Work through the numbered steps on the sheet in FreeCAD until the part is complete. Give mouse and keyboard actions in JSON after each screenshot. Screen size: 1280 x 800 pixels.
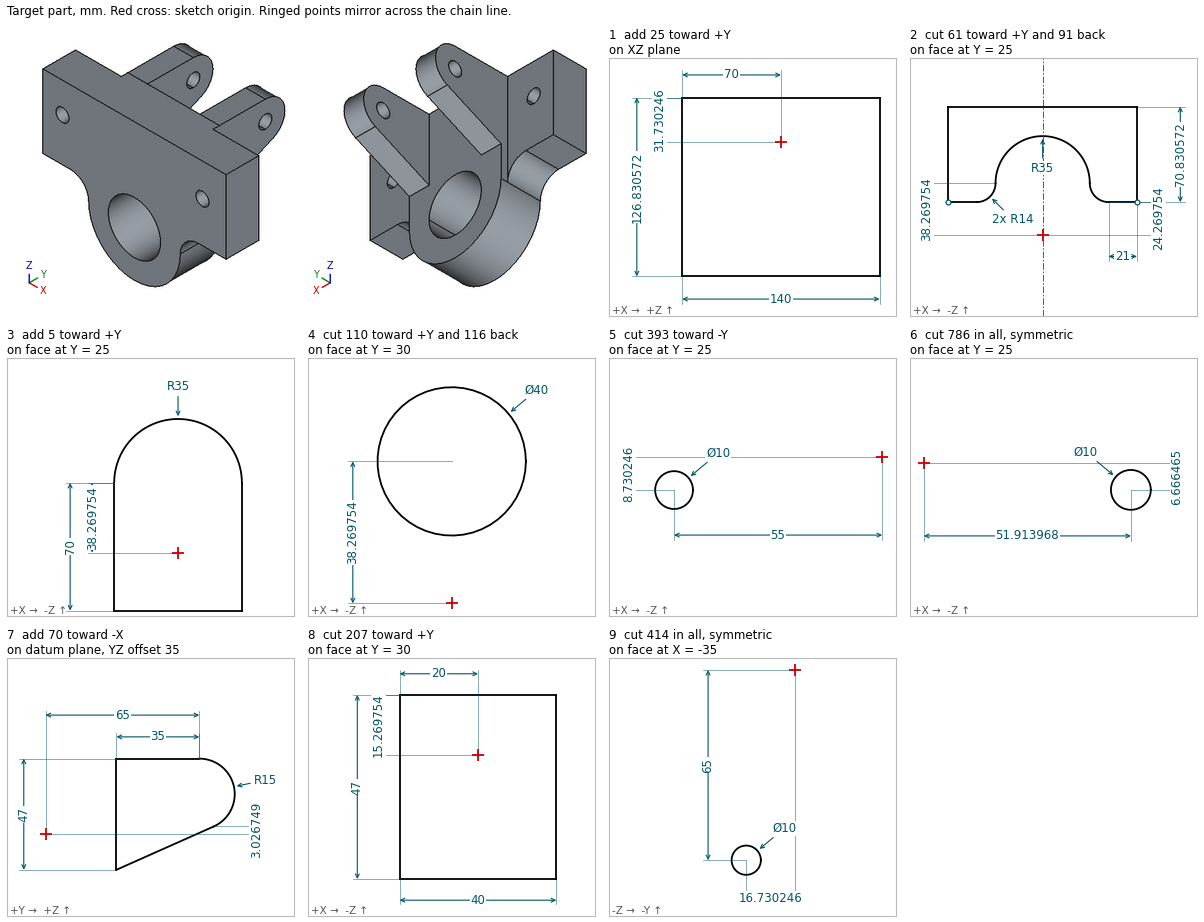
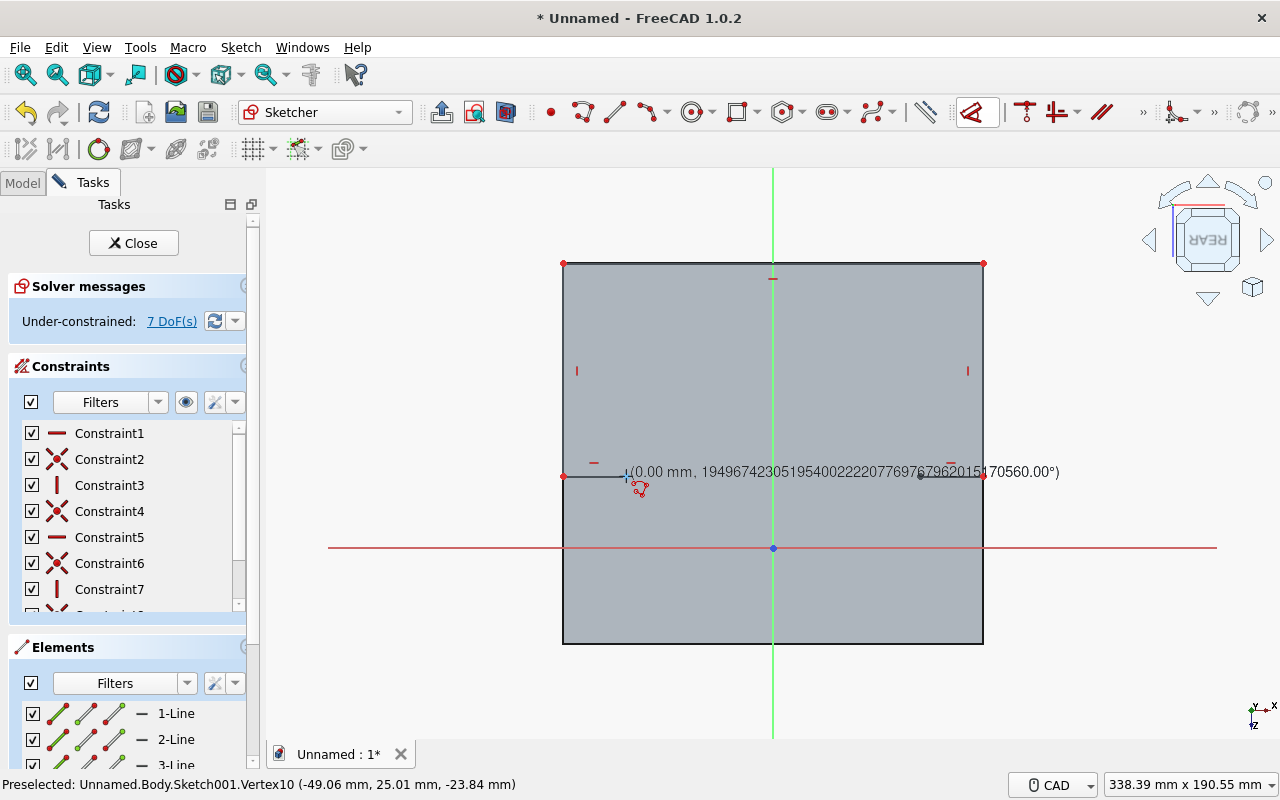
{"action": "left_click", "coordinate": [648, 112]}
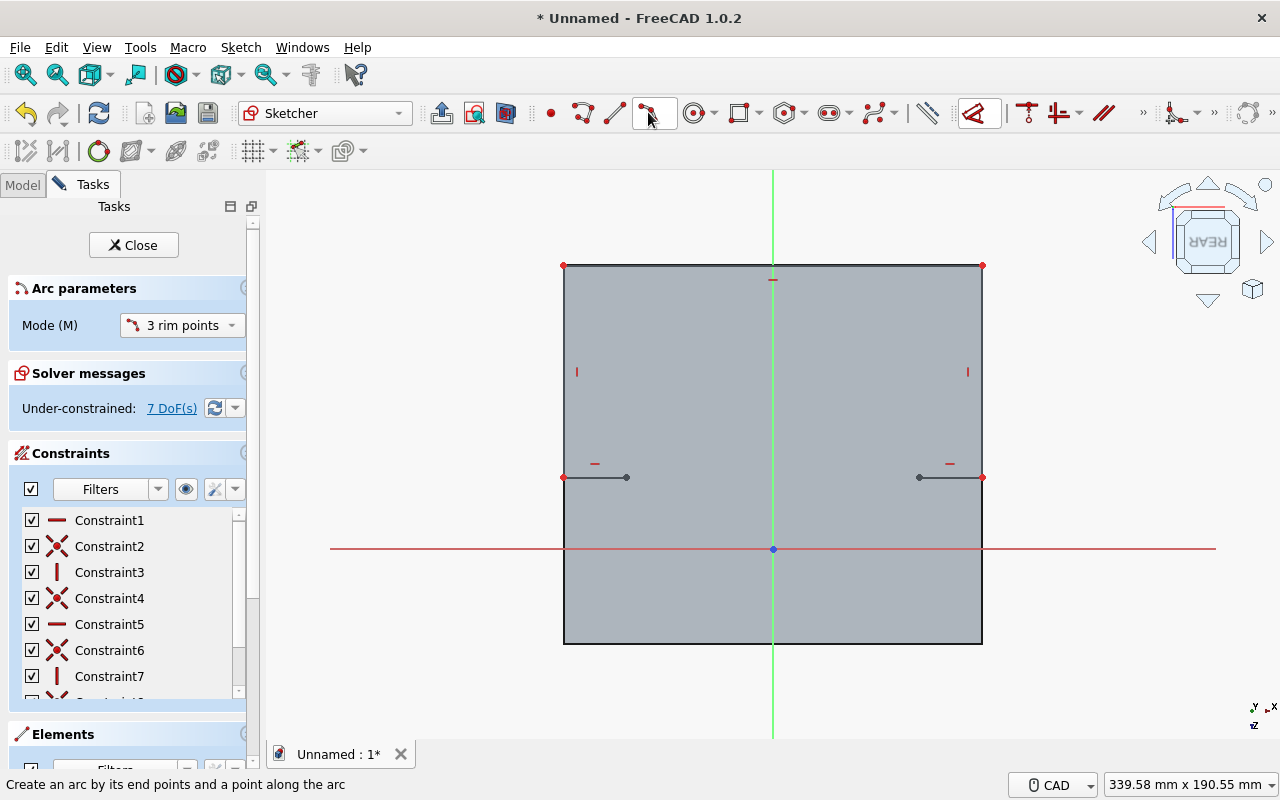
{"action": "left_click", "coordinate": [627, 478]}
{"action": "left_click", "coordinate": [668, 435]}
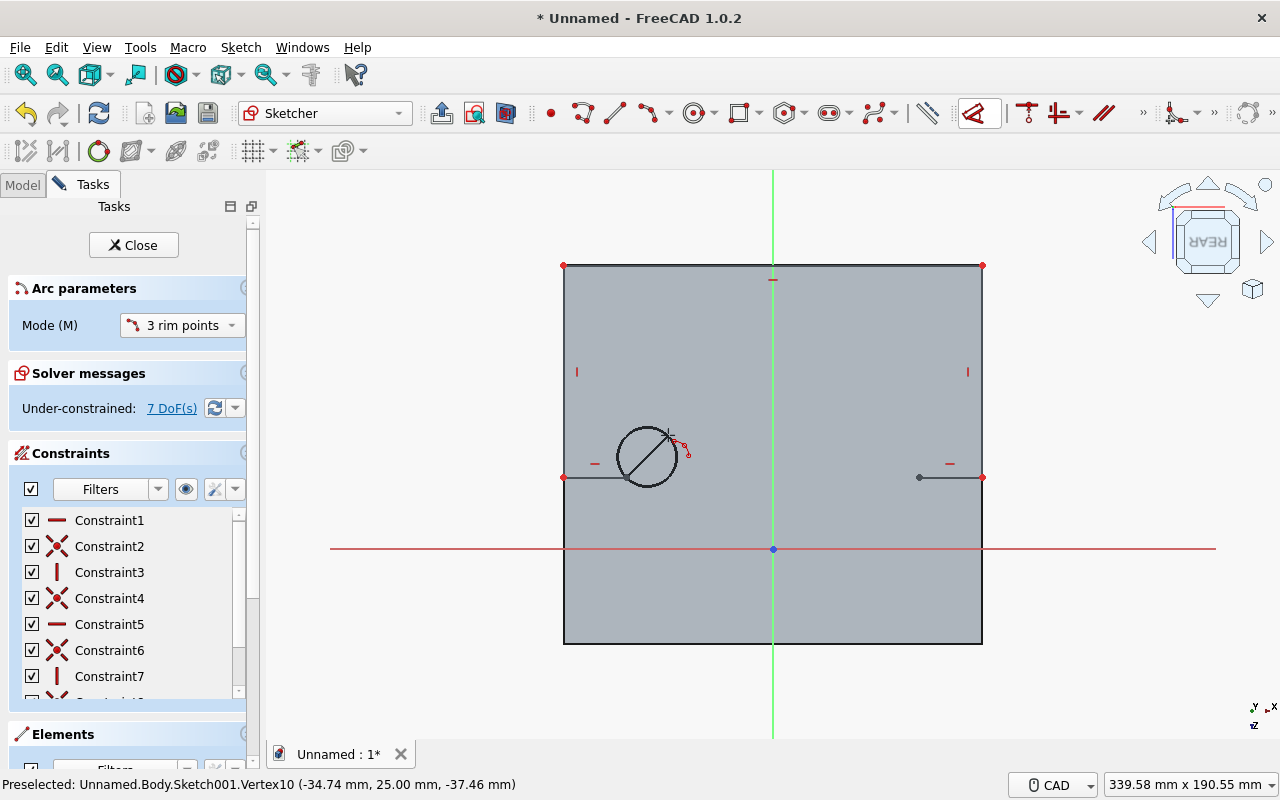
{"action": "scroll", "coordinate": [656, 464], "scroll_direction": "up", "scroll_amount": 2}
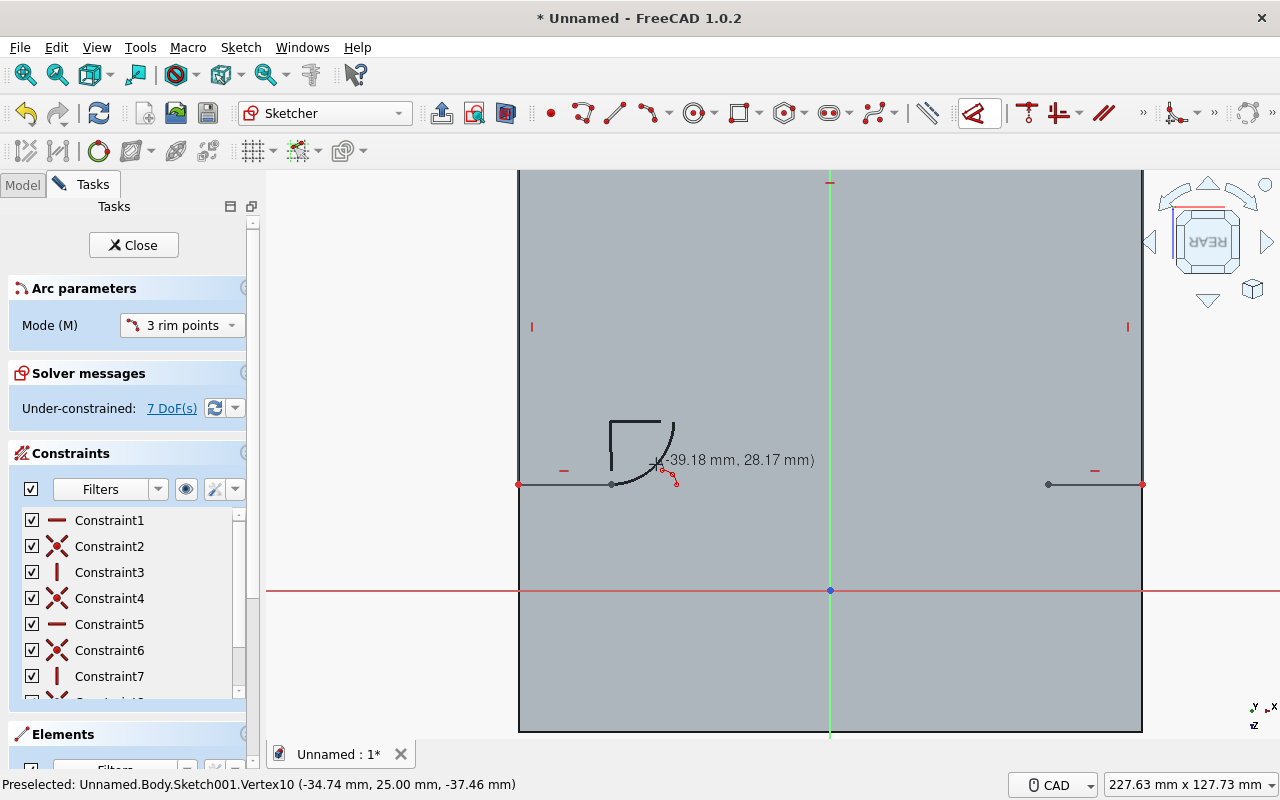
{"action": "left_click", "coordinate": [656, 464]}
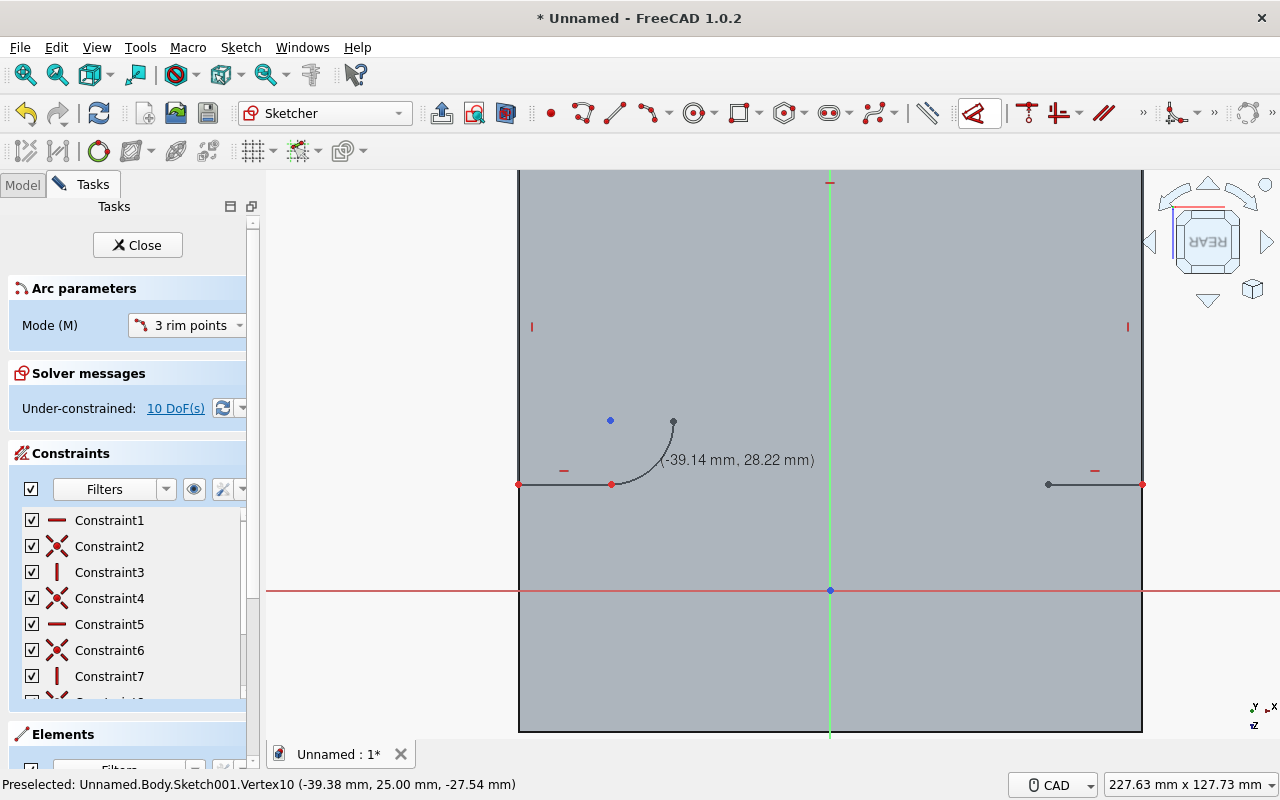
{"action": "left_click", "coordinate": [674, 422]}
{"action": "left_click", "coordinate": [986, 420]}
{"action": "left_click", "coordinate": [879, 272]}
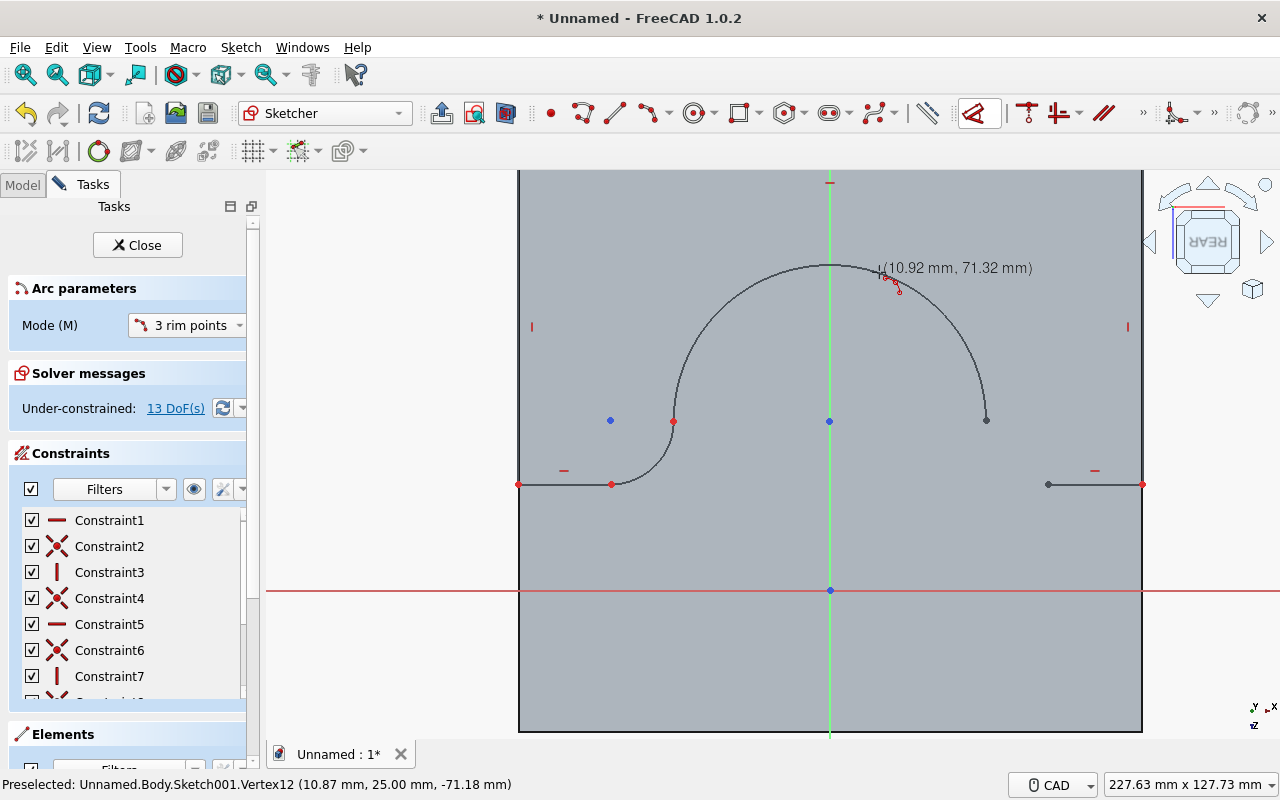
{"action": "left_click", "coordinate": [986, 421]}
{"action": "left_click", "coordinate": [1049, 485]}
{"action": "left_click", "coordinate": [1005, 464]}
{"action": "key", "text": "Escape"}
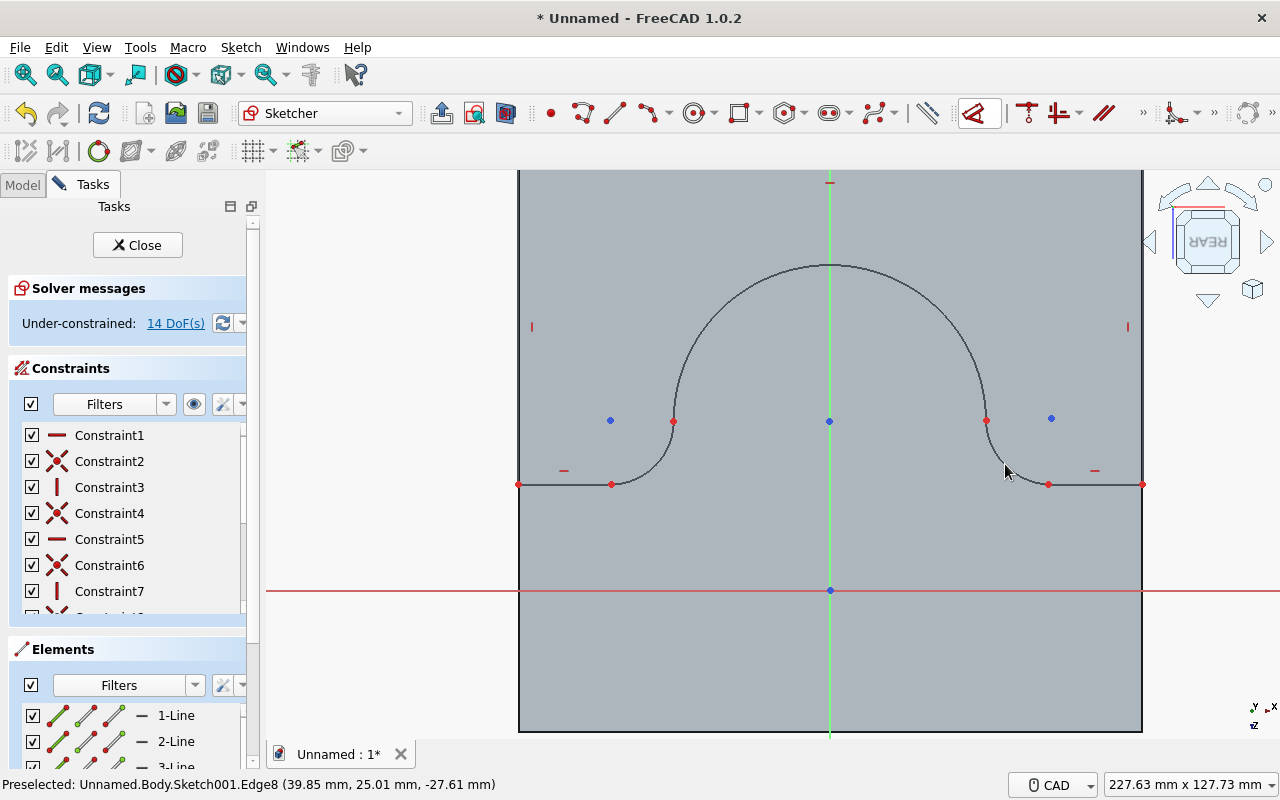
{"action": "left_click", "coordinate": [1077, 485]}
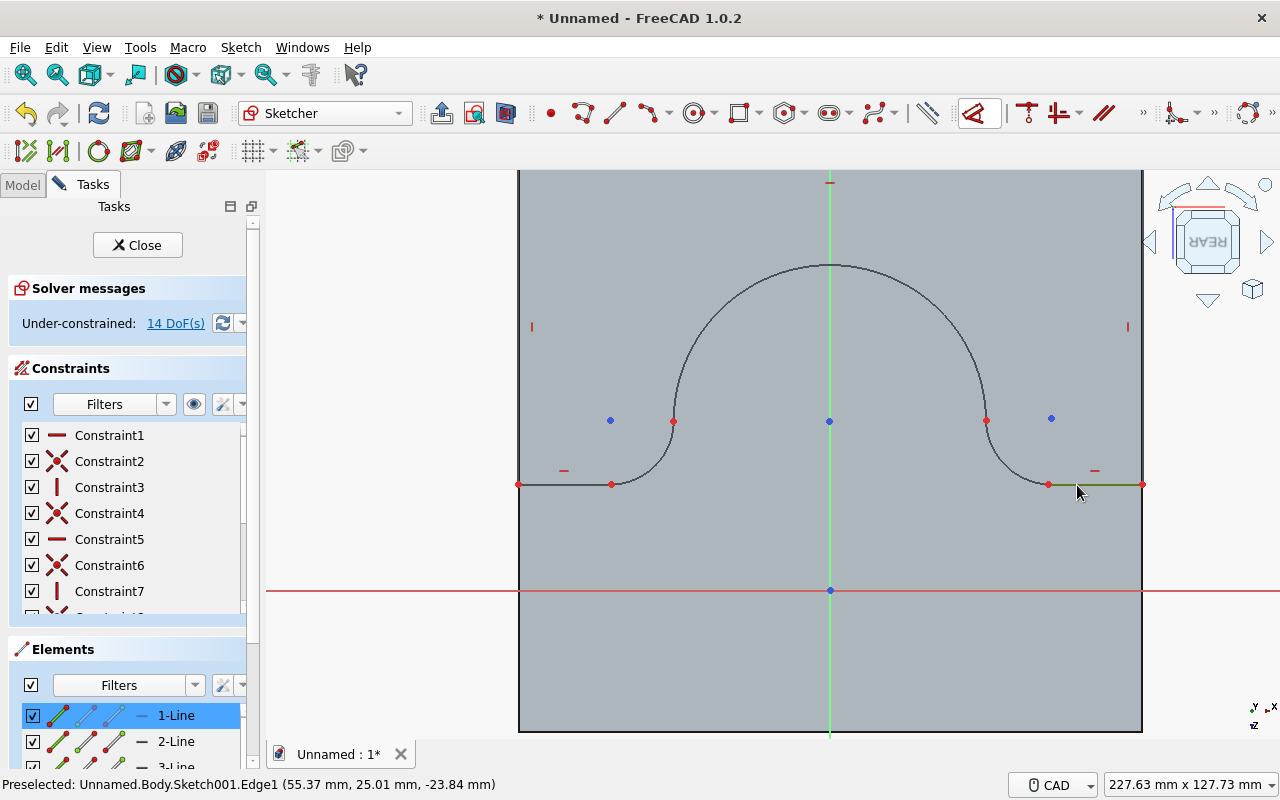
{"action": "left_click", "coordinate": [993, 449]}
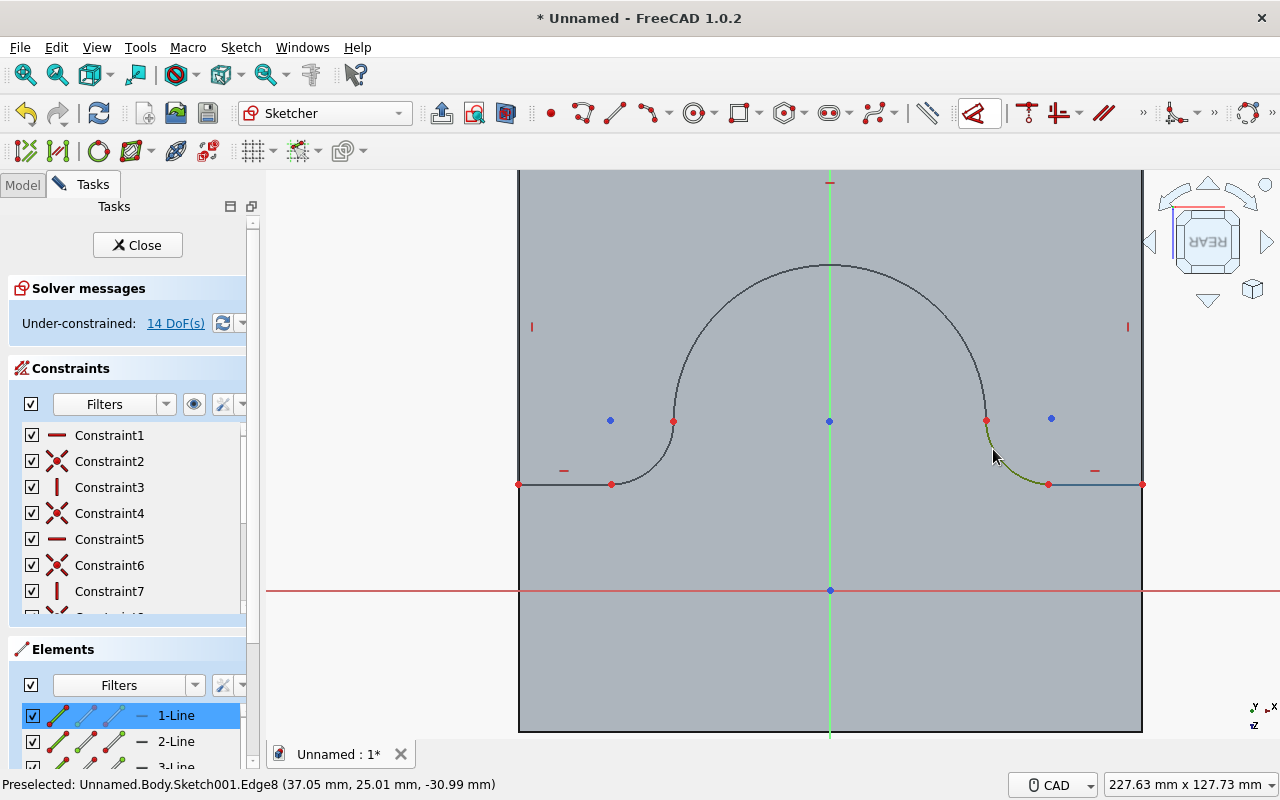
{"action": "key", "text": "t"}